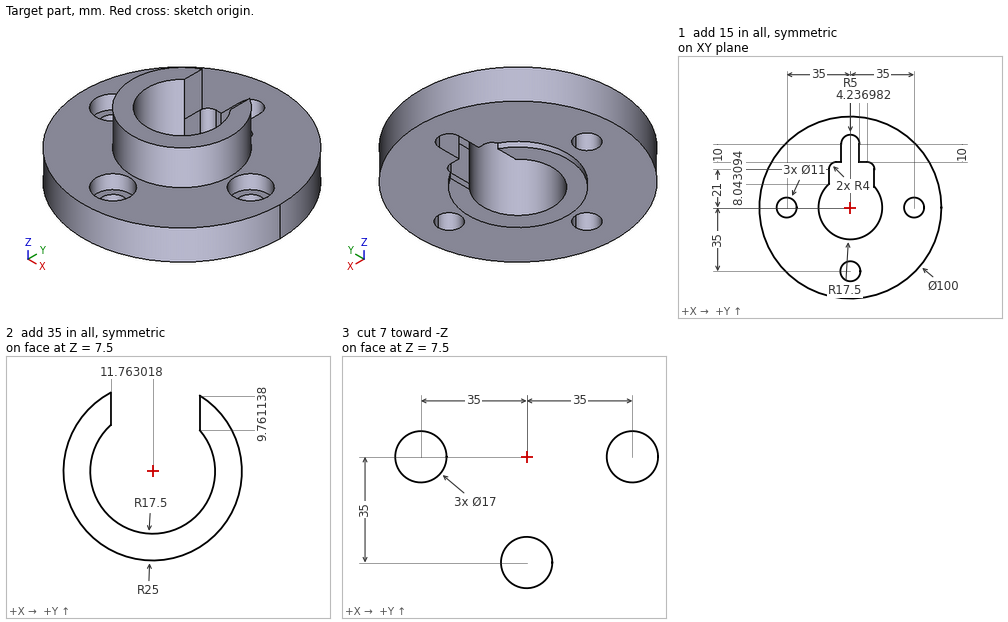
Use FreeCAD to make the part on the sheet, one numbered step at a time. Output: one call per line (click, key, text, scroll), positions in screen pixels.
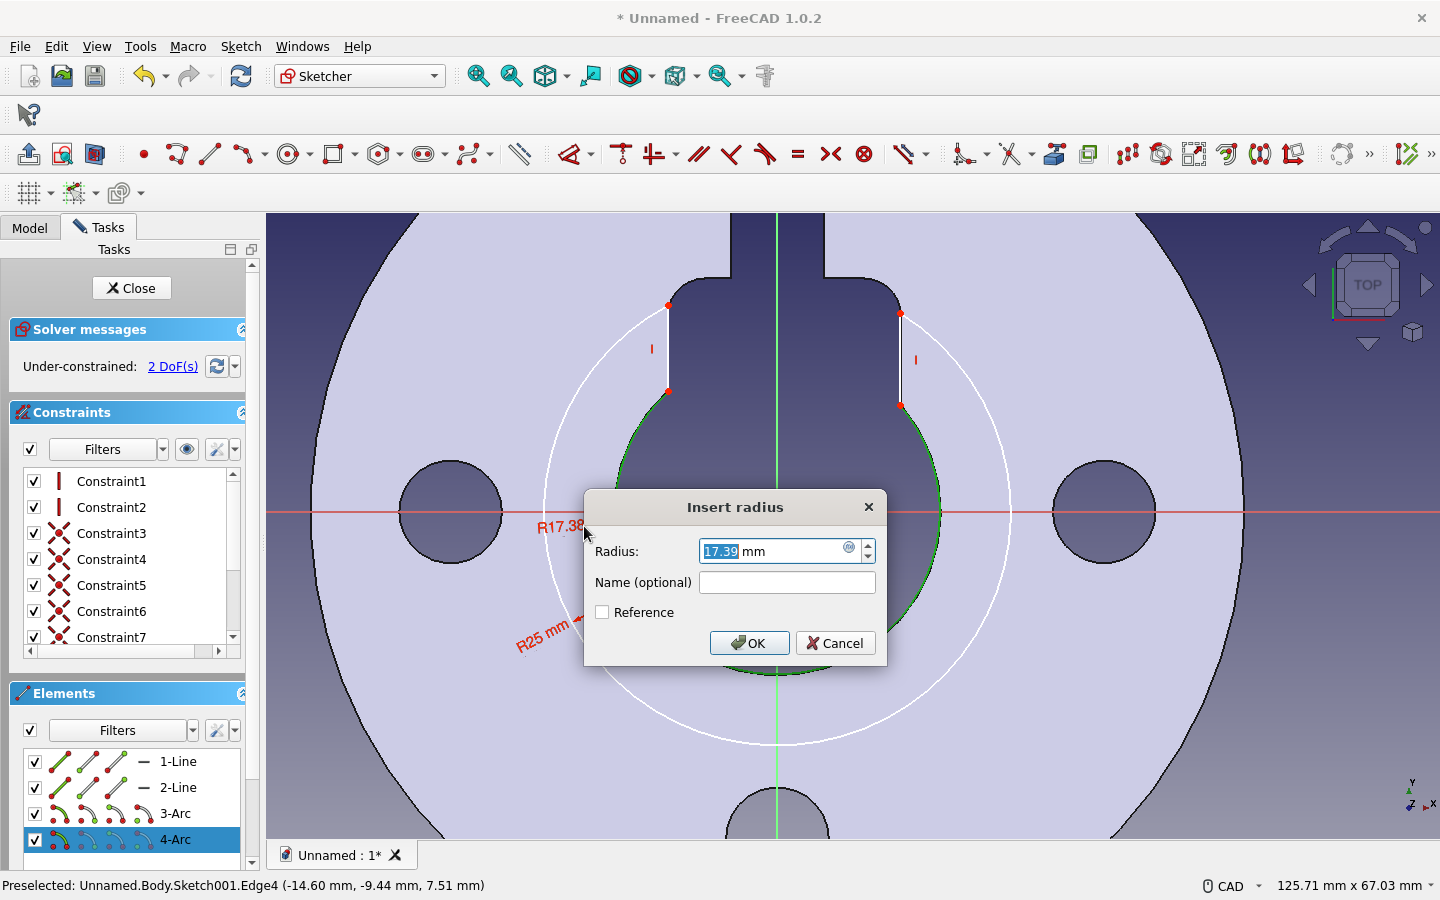
text(17.5)
key(Return)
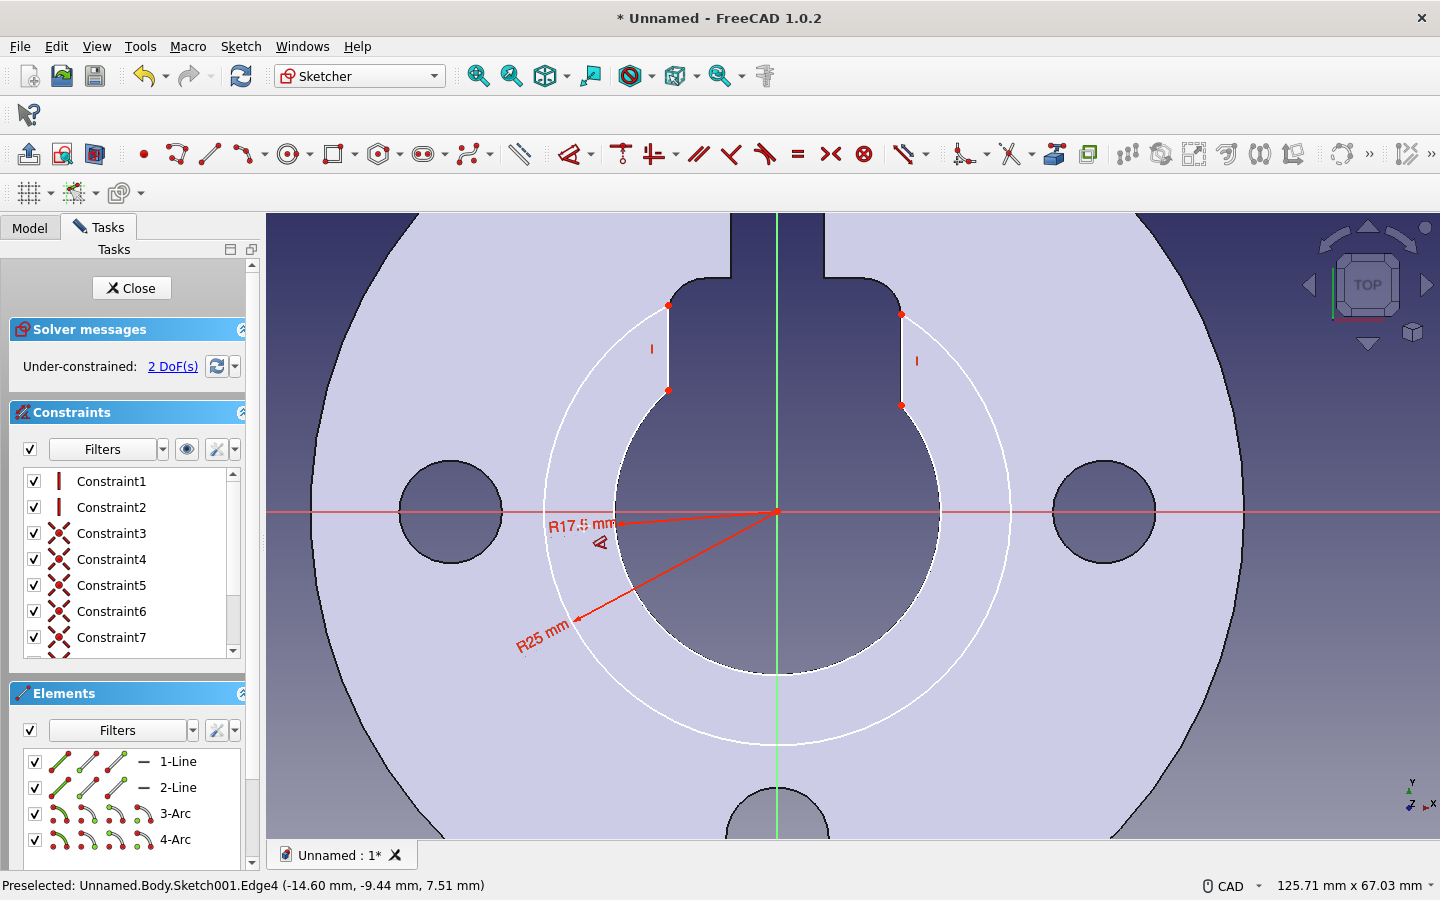
click(902, 342)
click(936, 360)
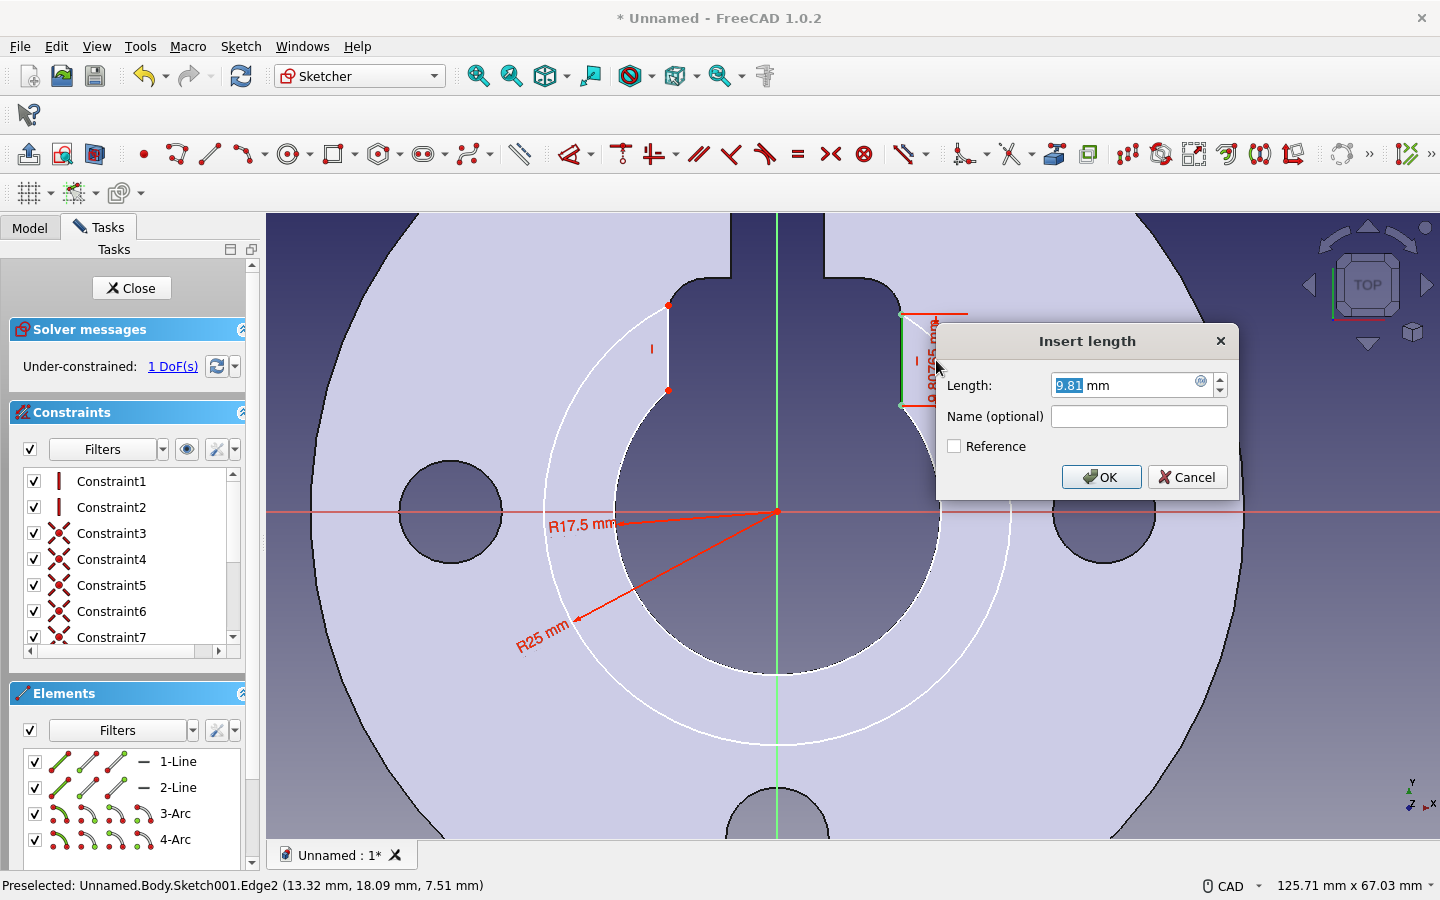
text(9.761138)
key(Return)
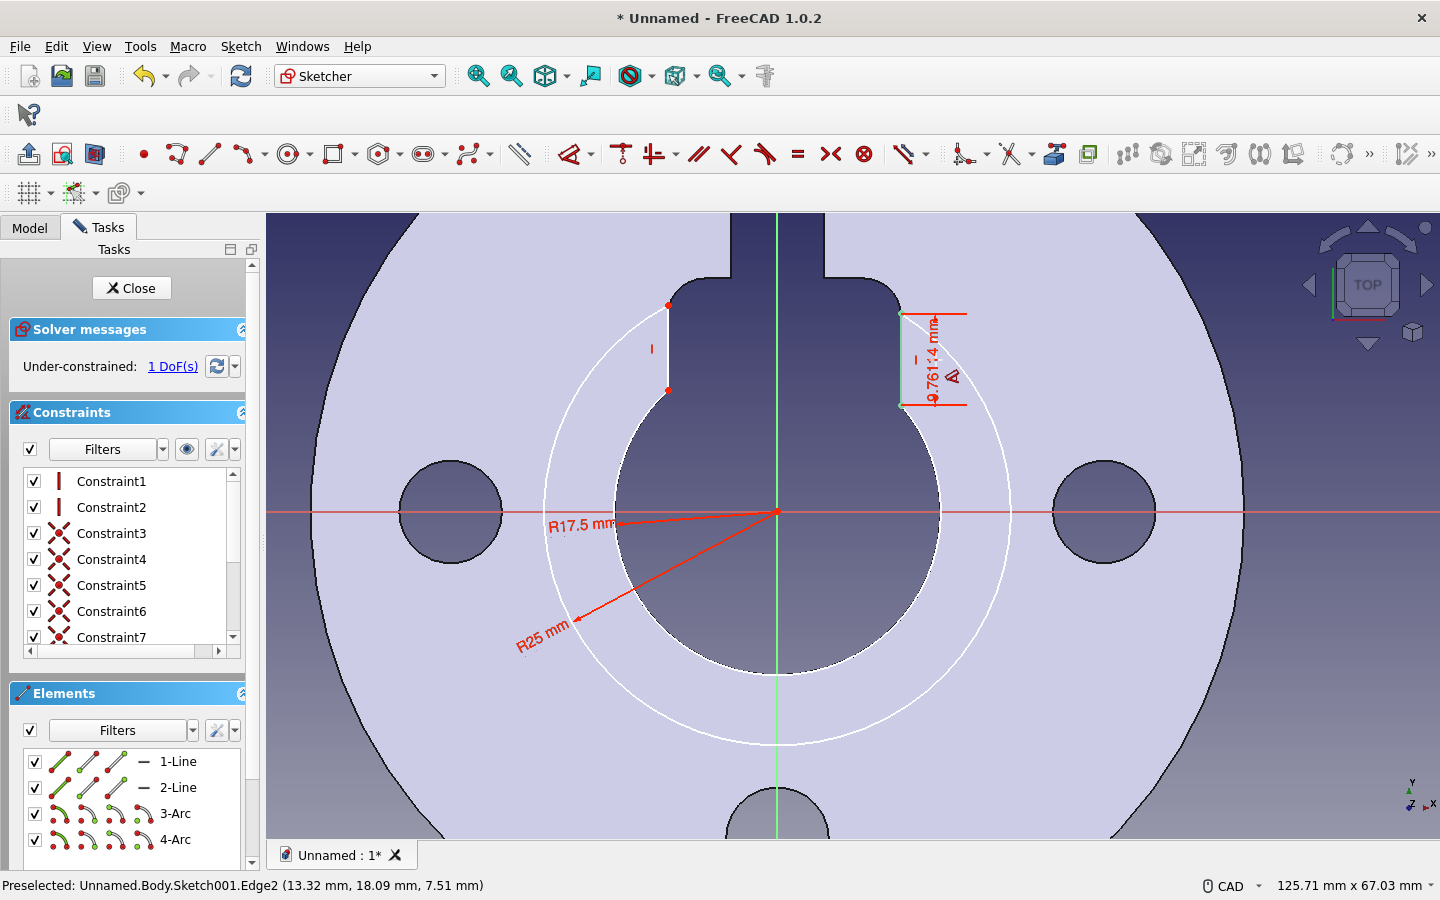
click(668, 391)
click(723, 357)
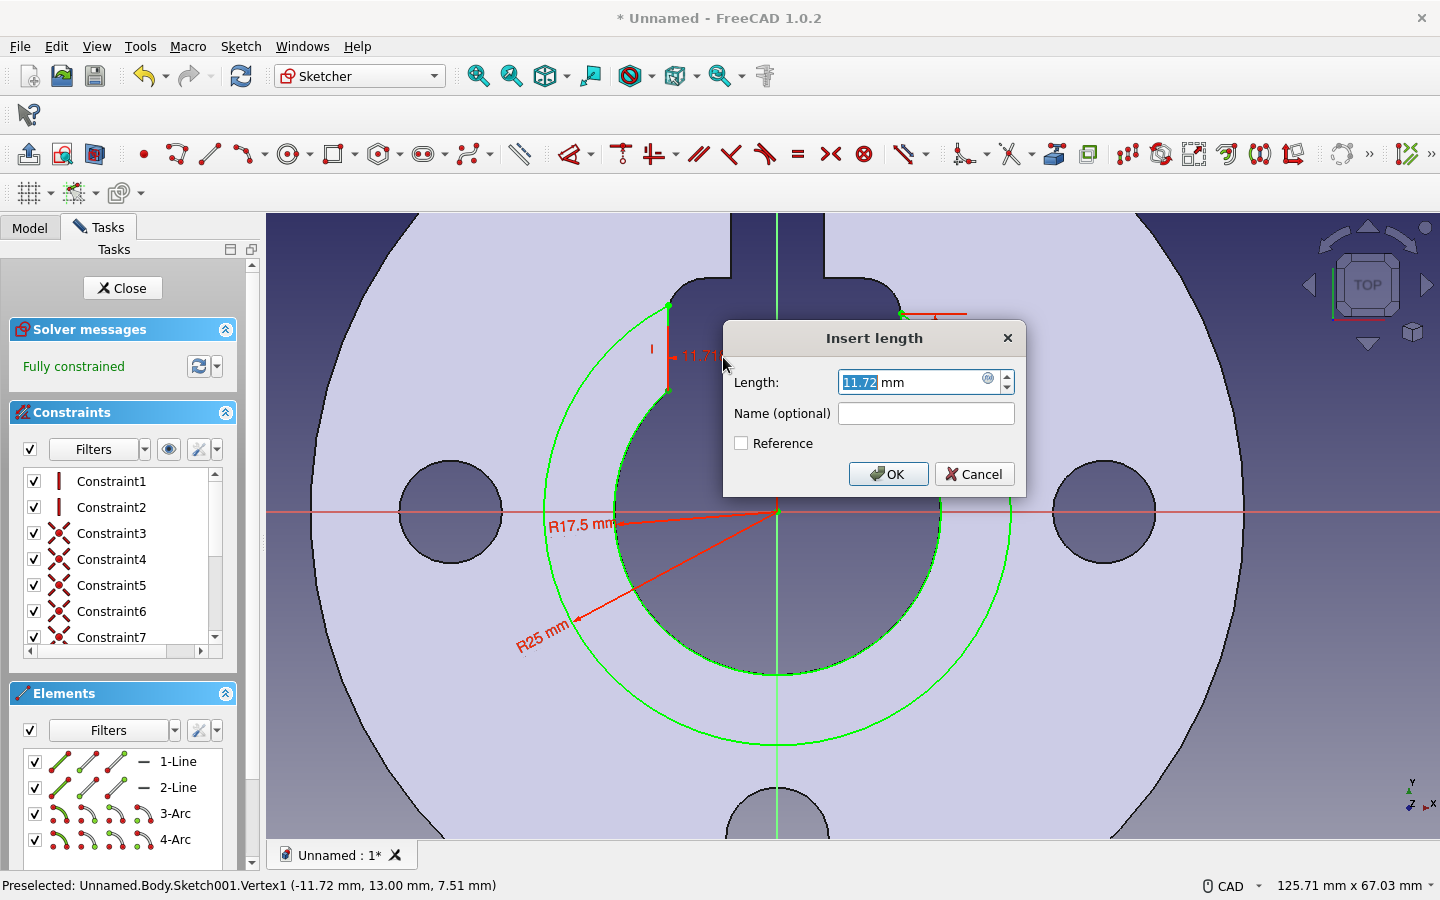
text(11.763018)
key(Return)
key(Escape)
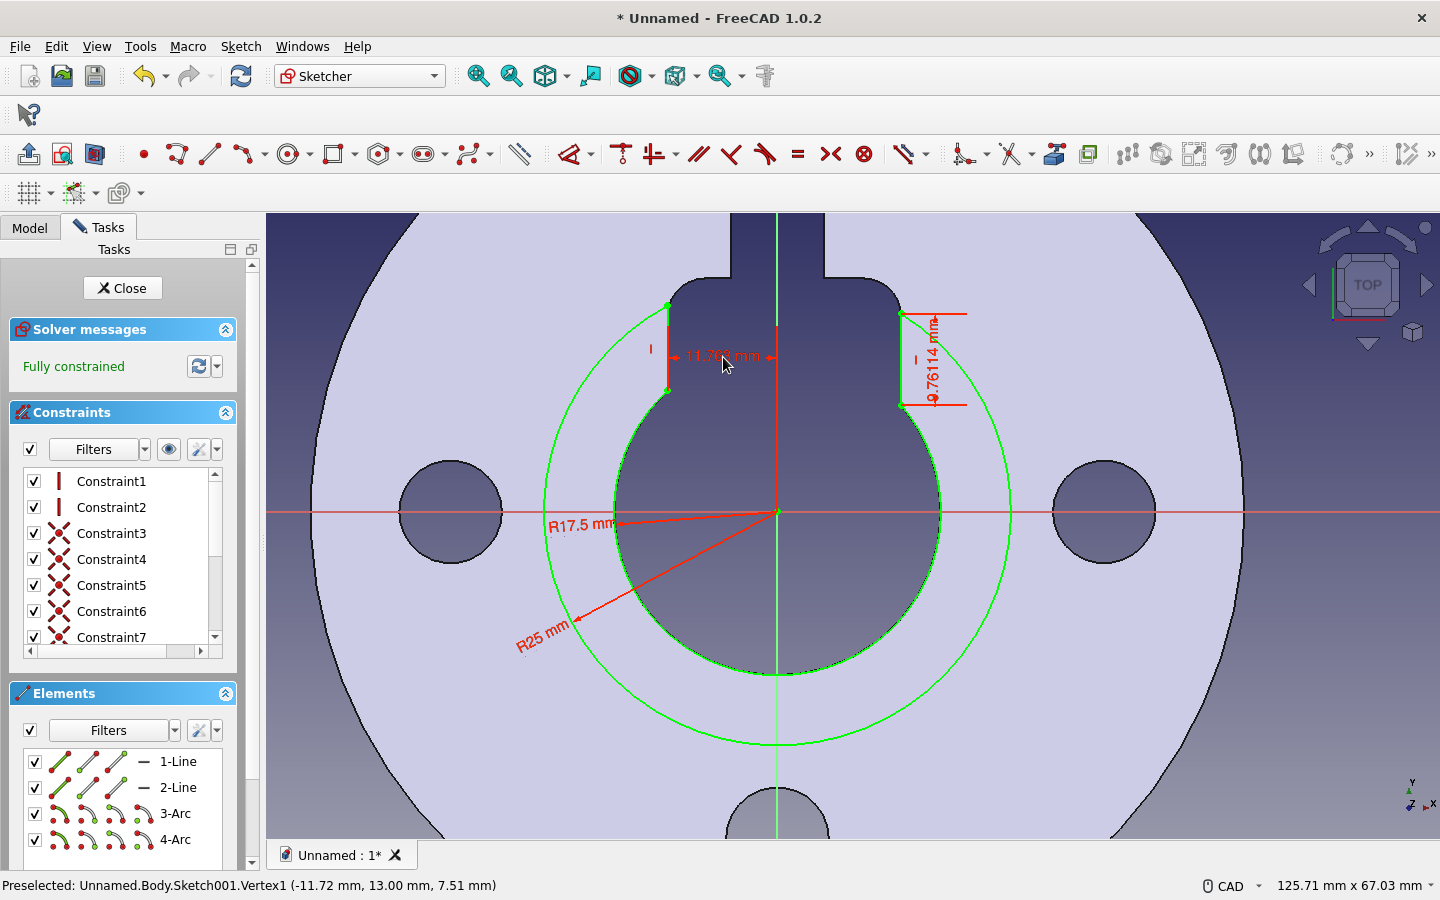
click(123, 288)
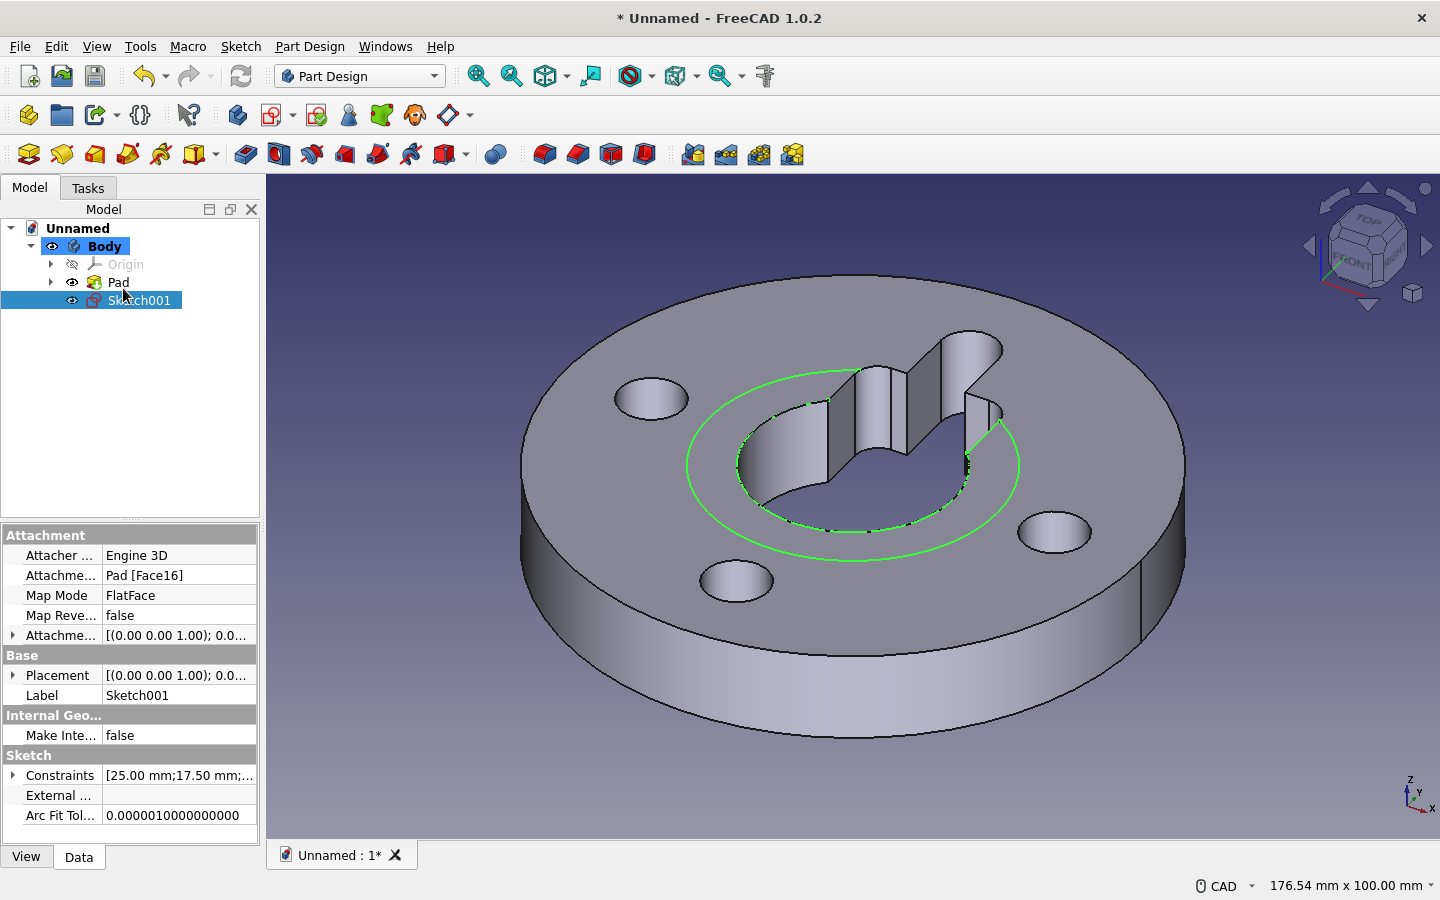
click(29, 154)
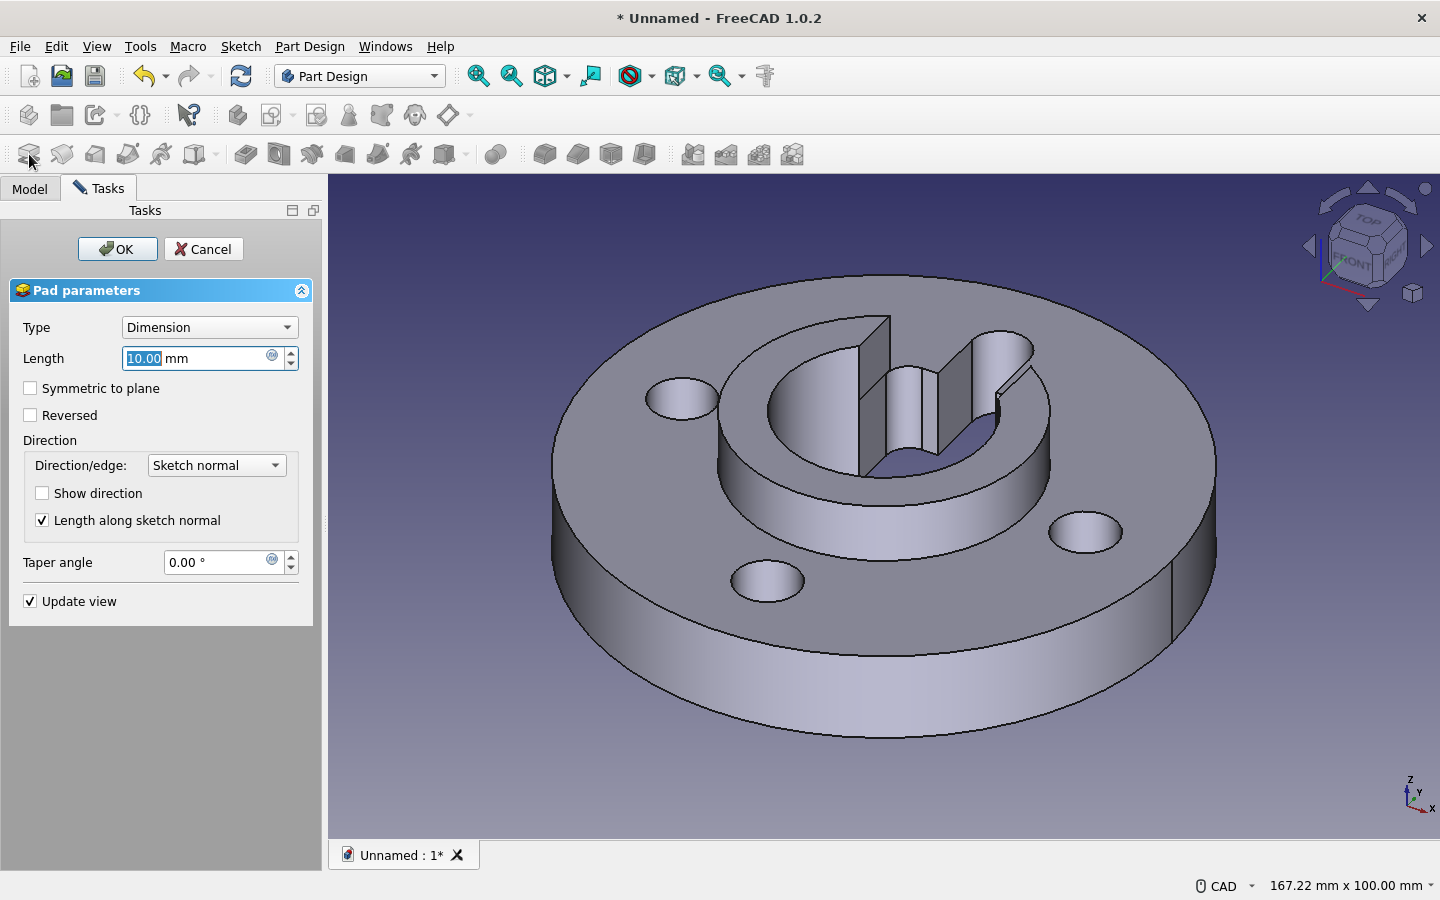
text(35)
key(Tab)